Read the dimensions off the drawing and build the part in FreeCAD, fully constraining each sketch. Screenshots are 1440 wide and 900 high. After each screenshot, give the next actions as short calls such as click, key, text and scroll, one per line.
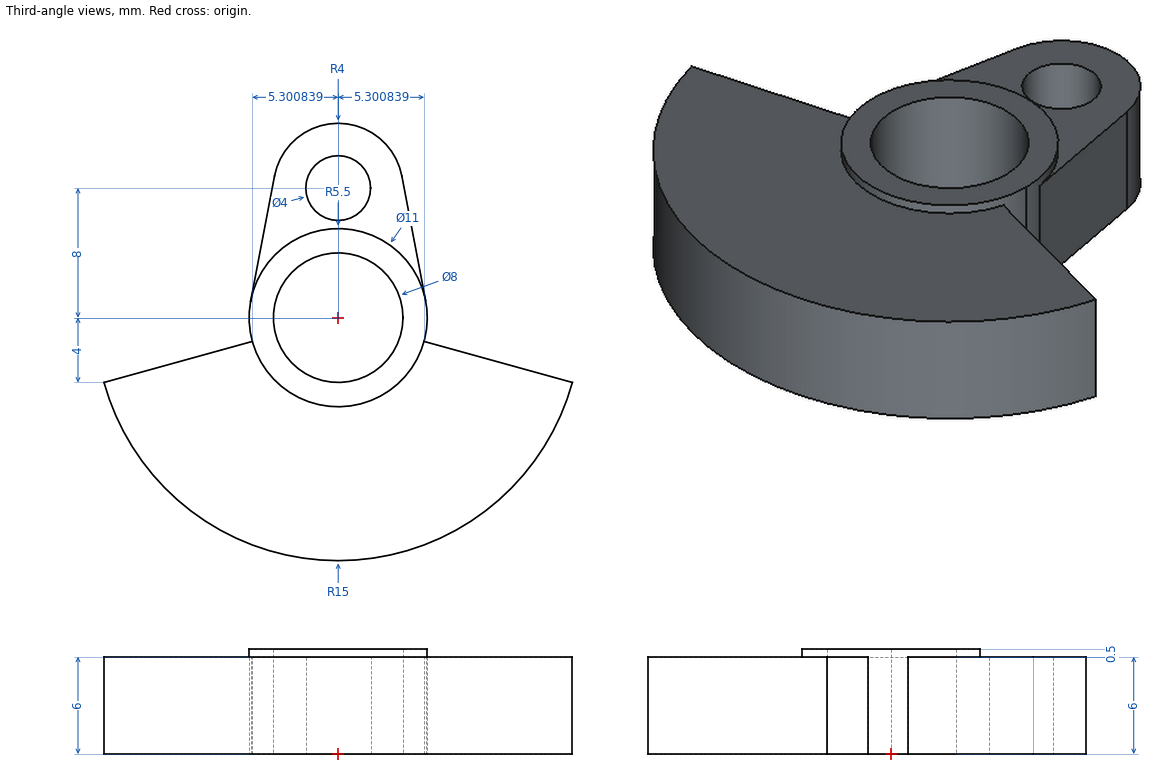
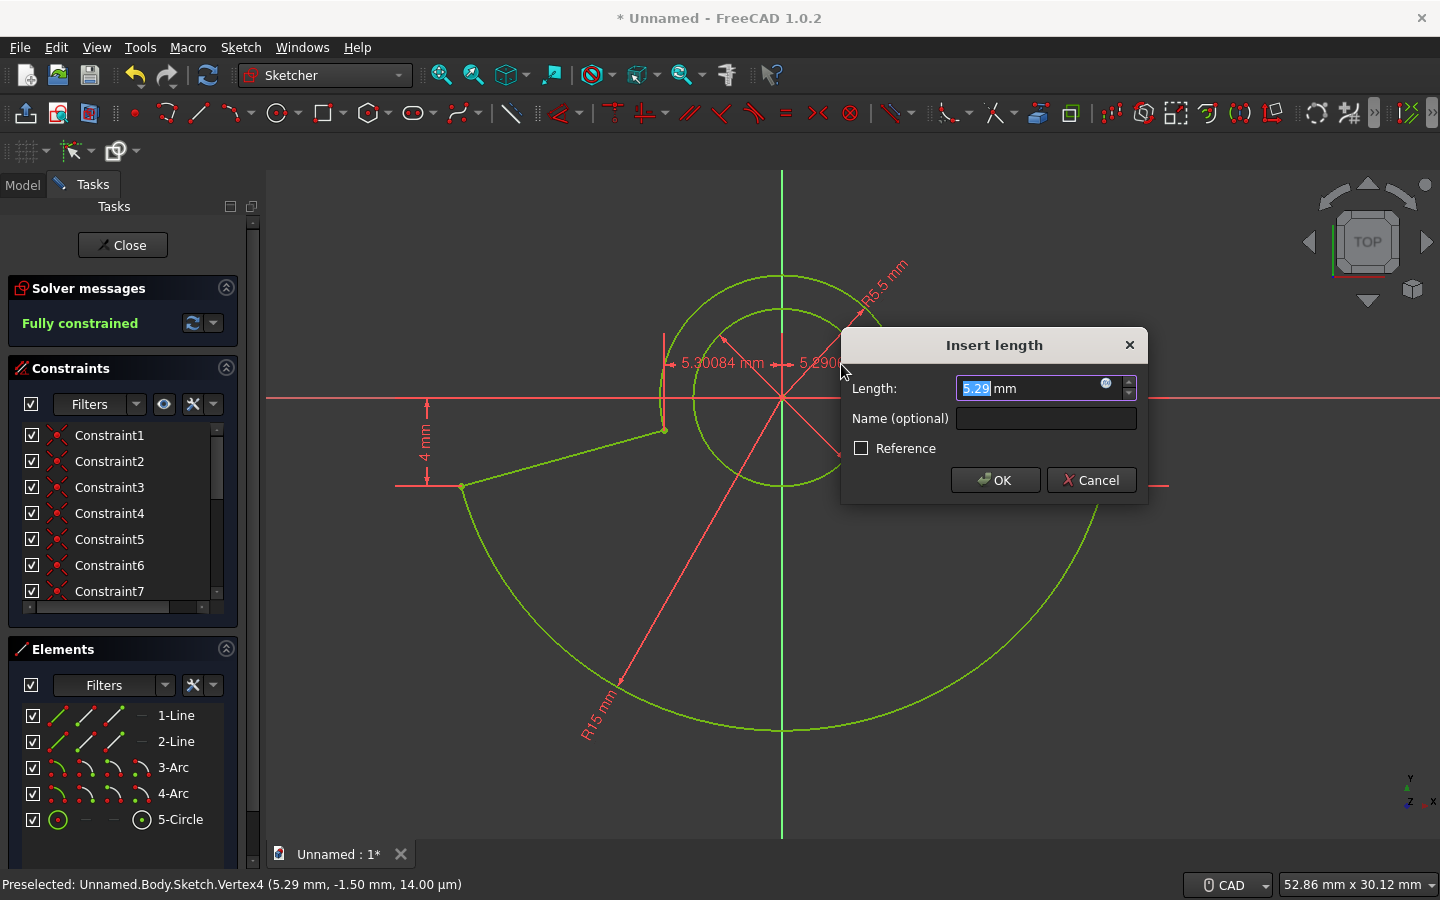
text(5.300839)
key(Return)
key(Escape)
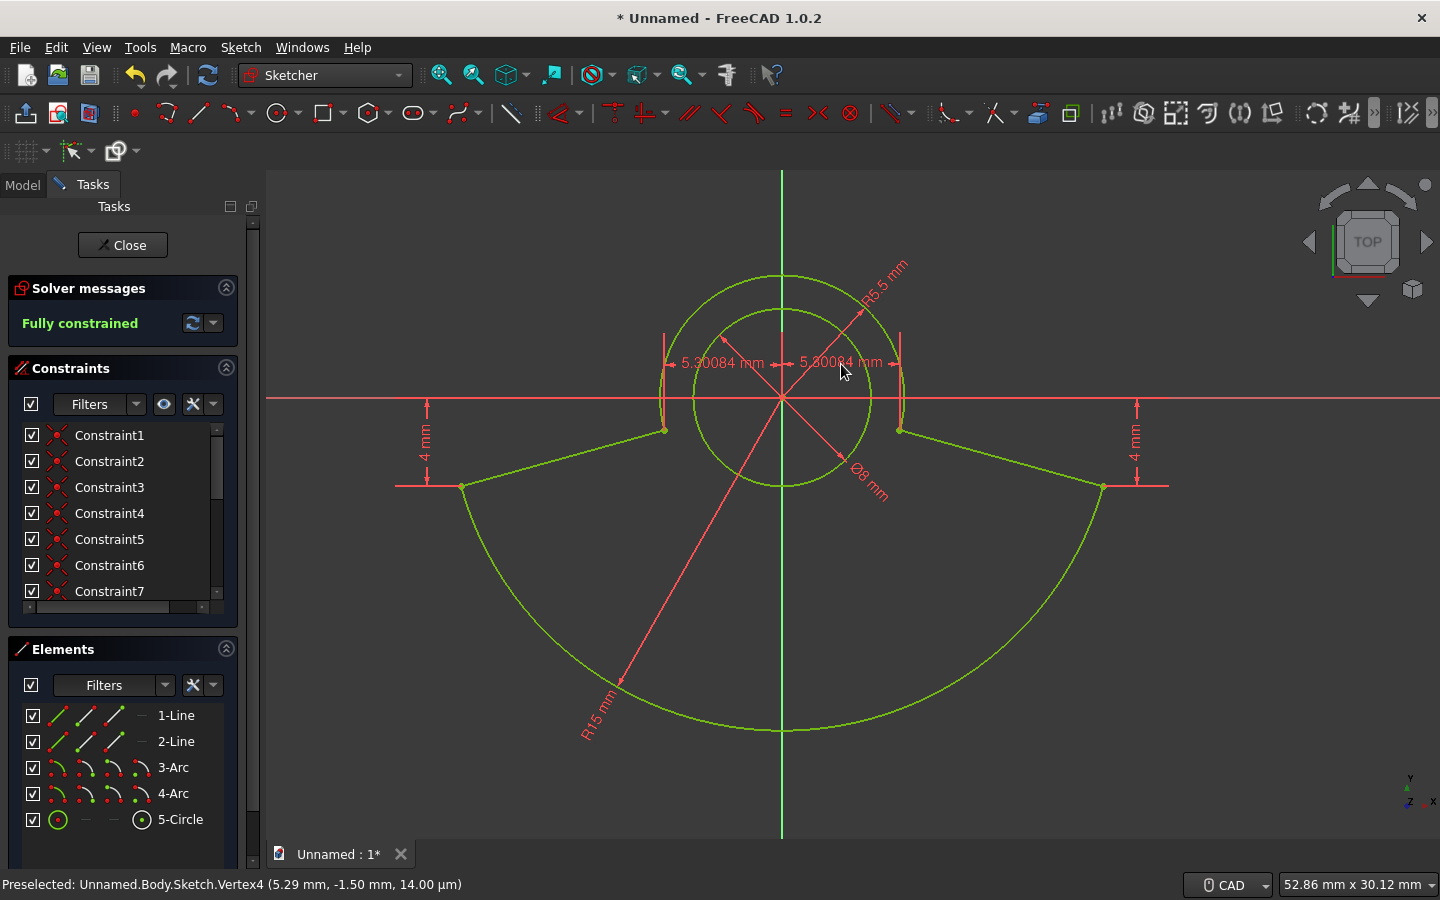
click(123, 245)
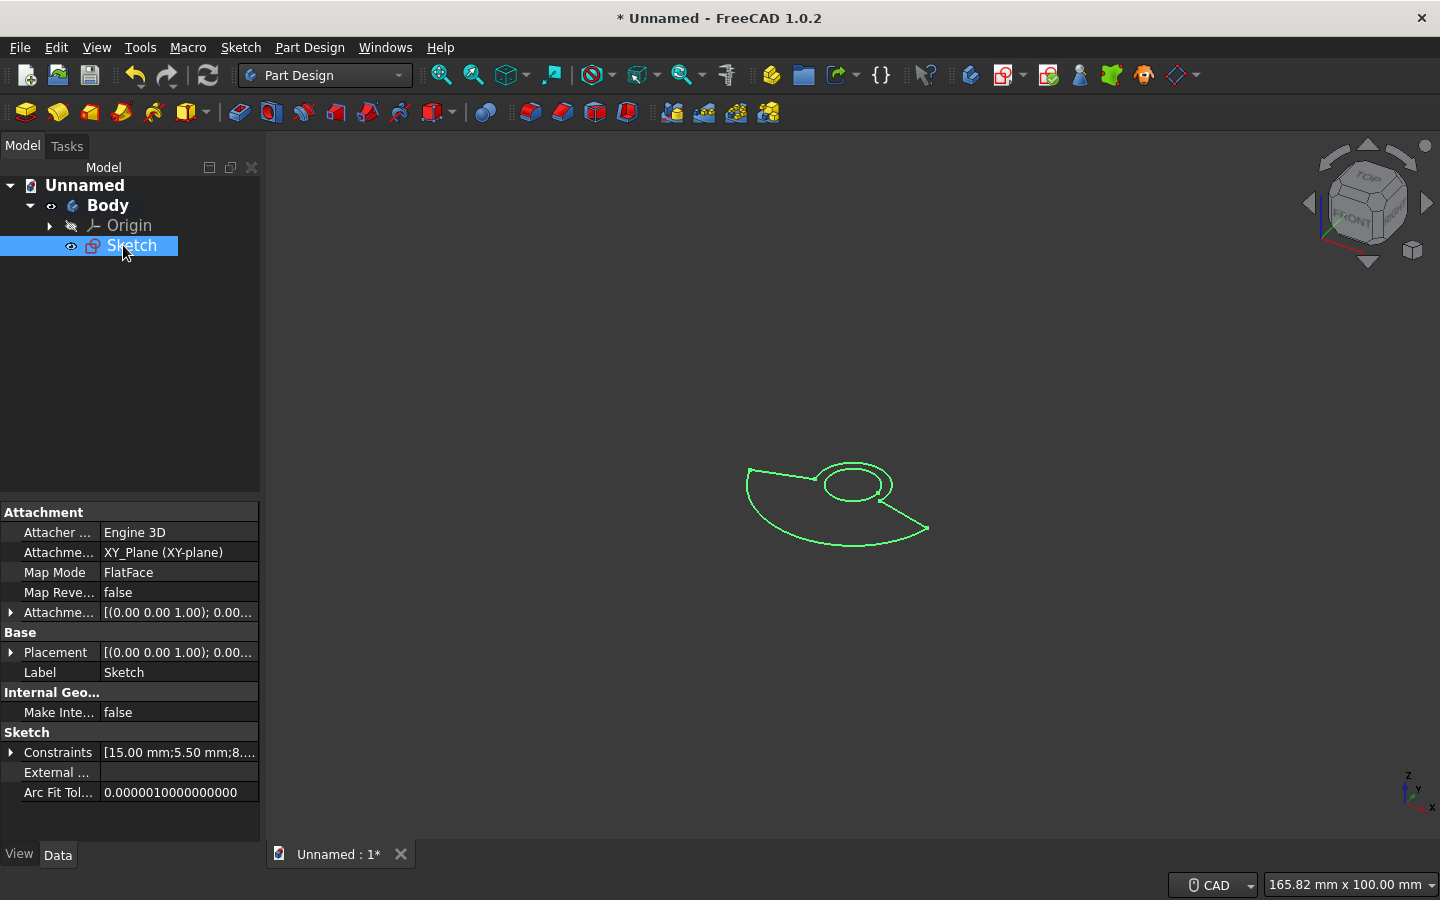
click(26, 112)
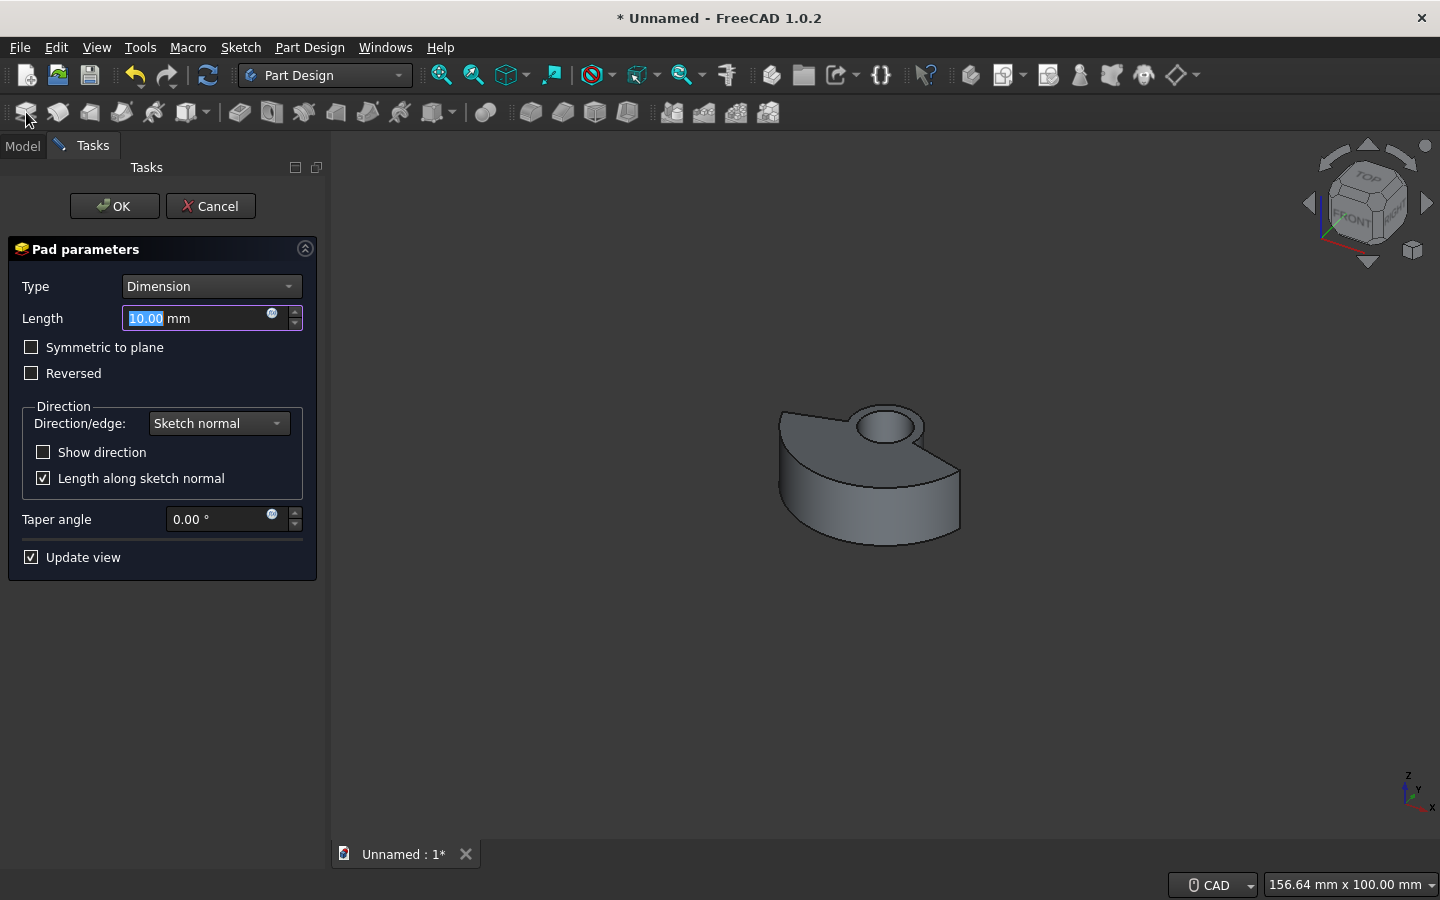
text(6)
key(Tab)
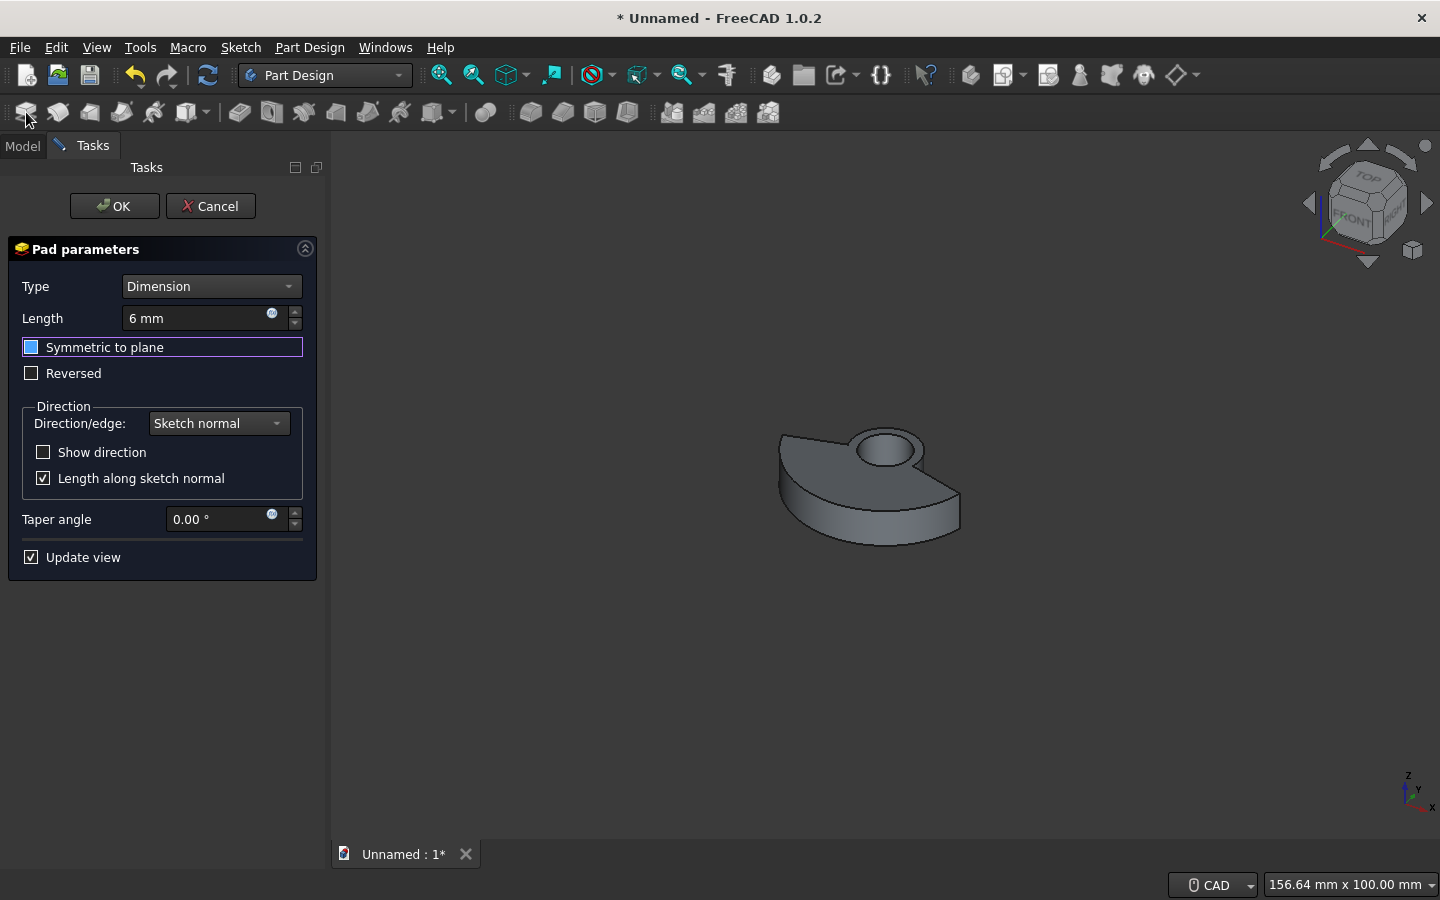
click(115, 206)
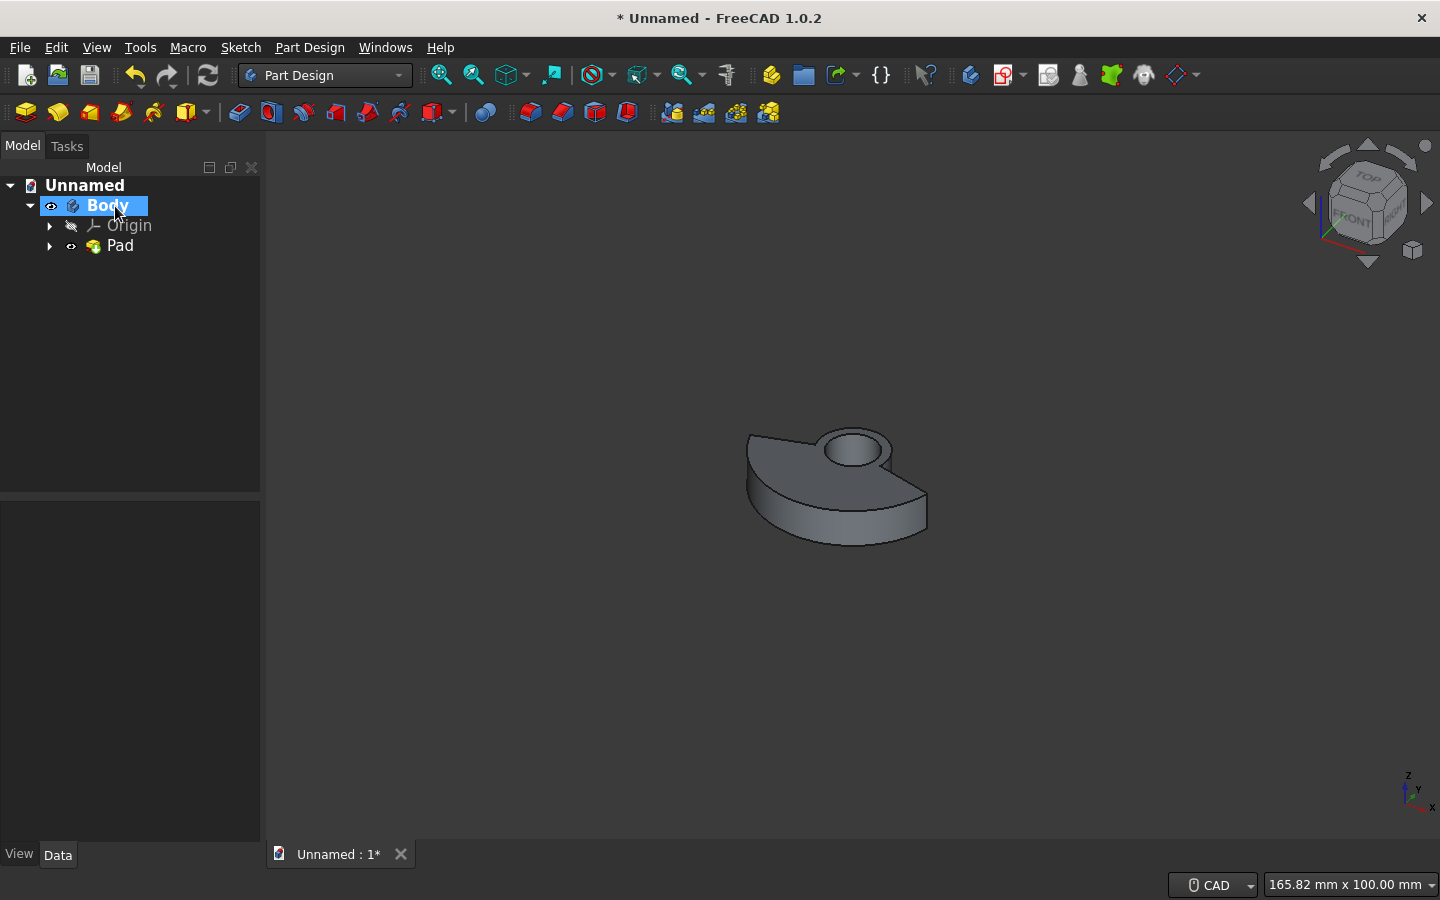
key(v)
key(f)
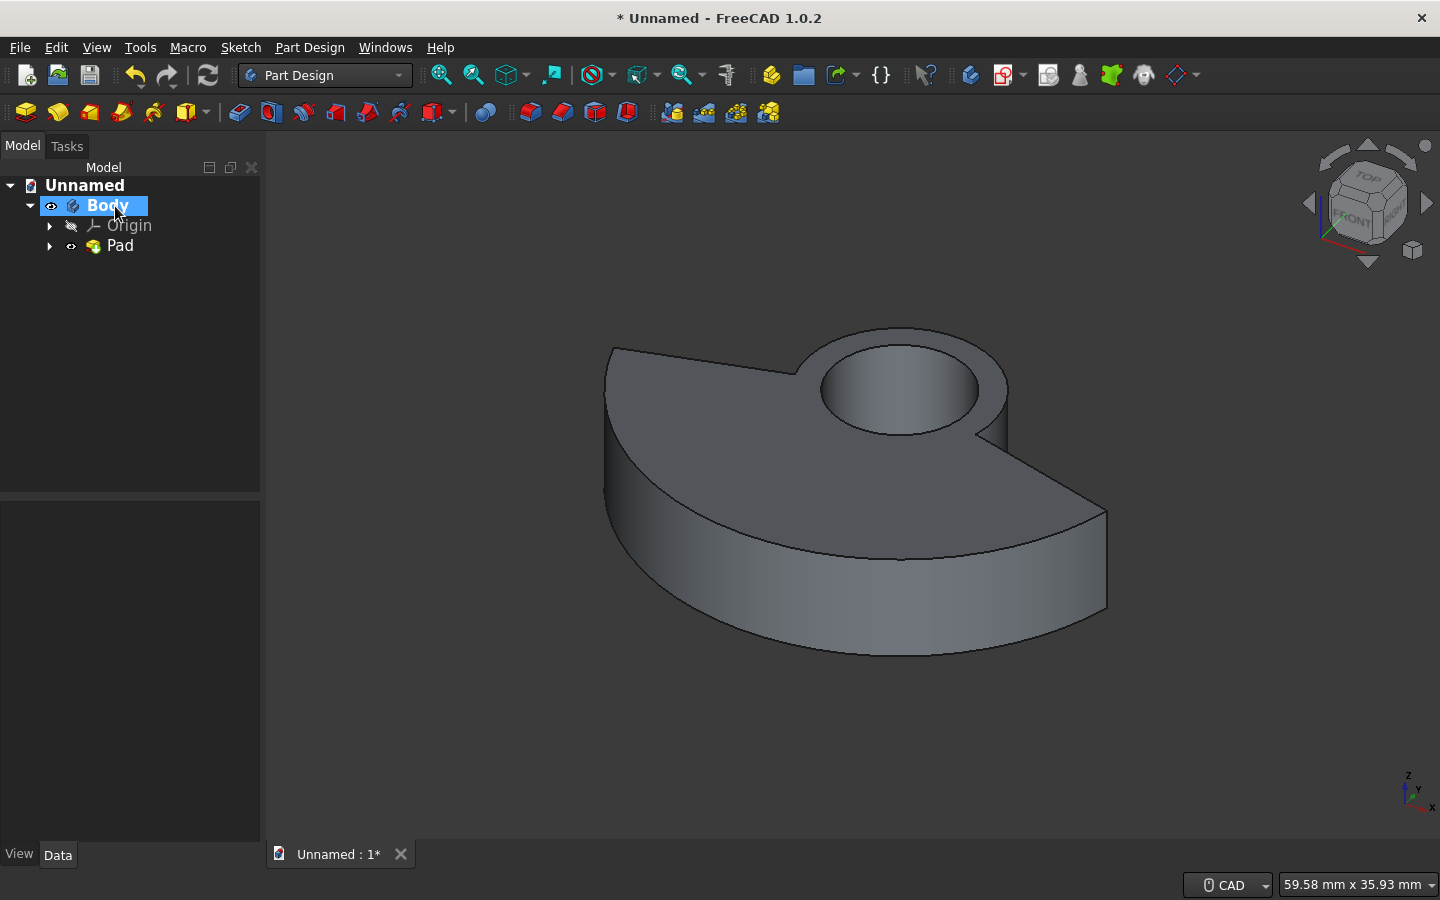
click(1004, 76)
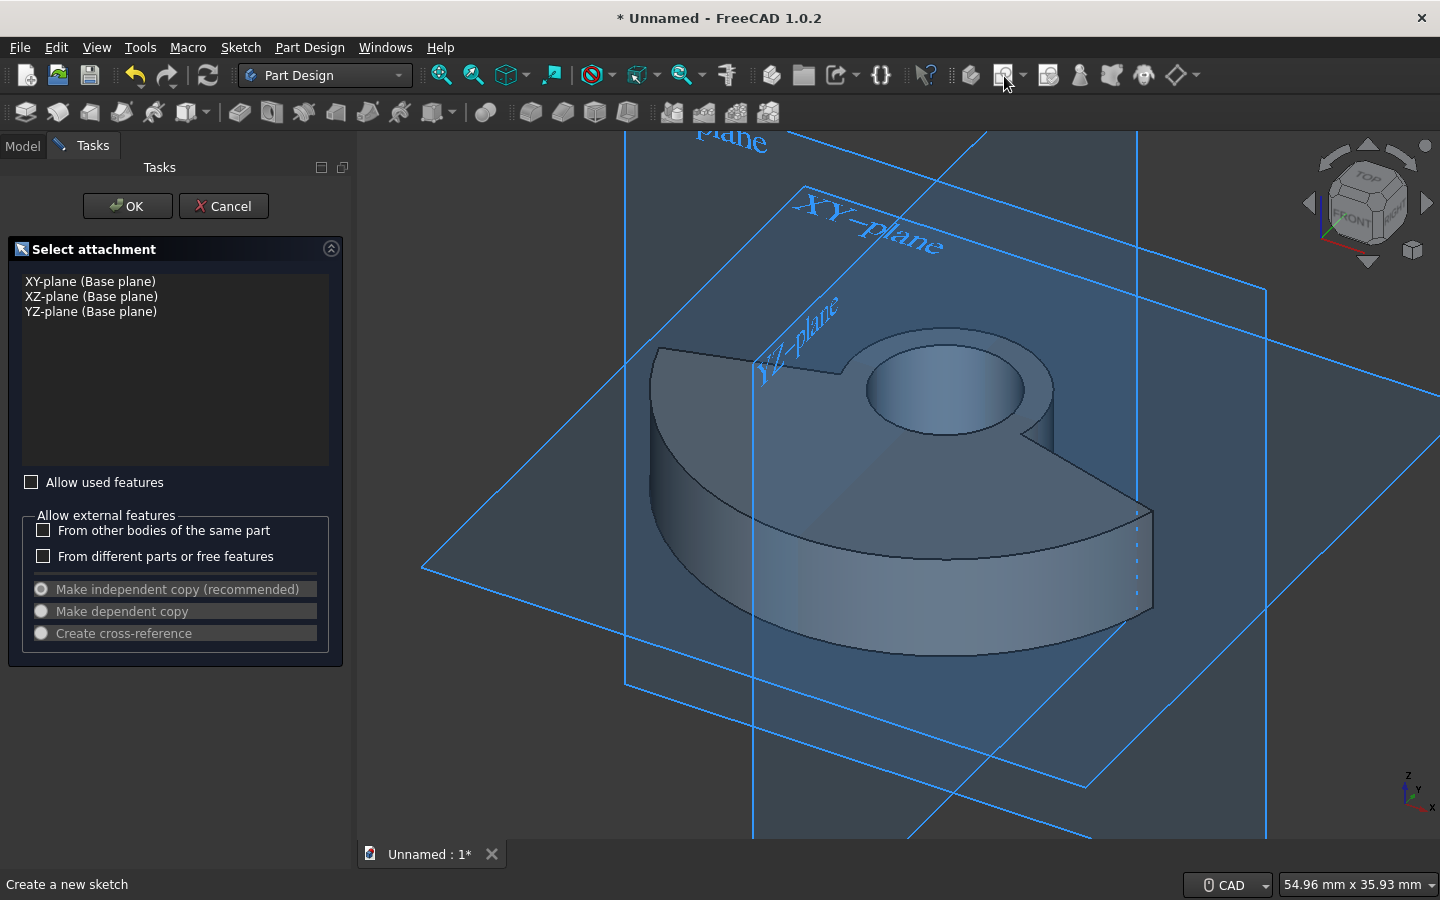
click(82, 282)